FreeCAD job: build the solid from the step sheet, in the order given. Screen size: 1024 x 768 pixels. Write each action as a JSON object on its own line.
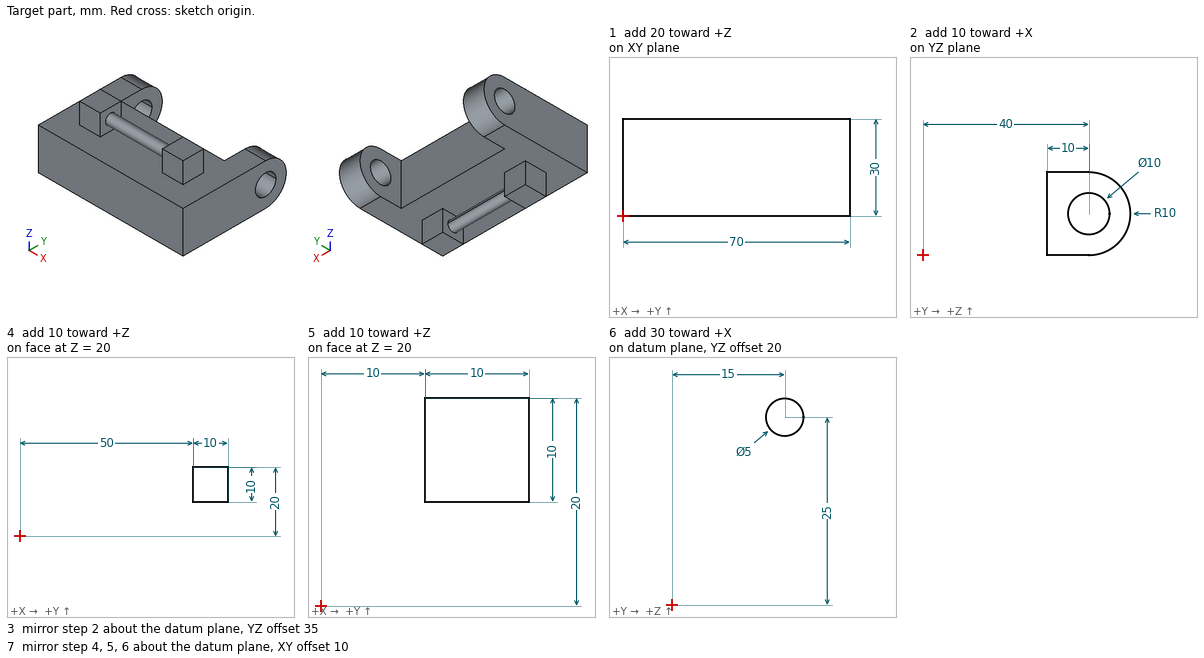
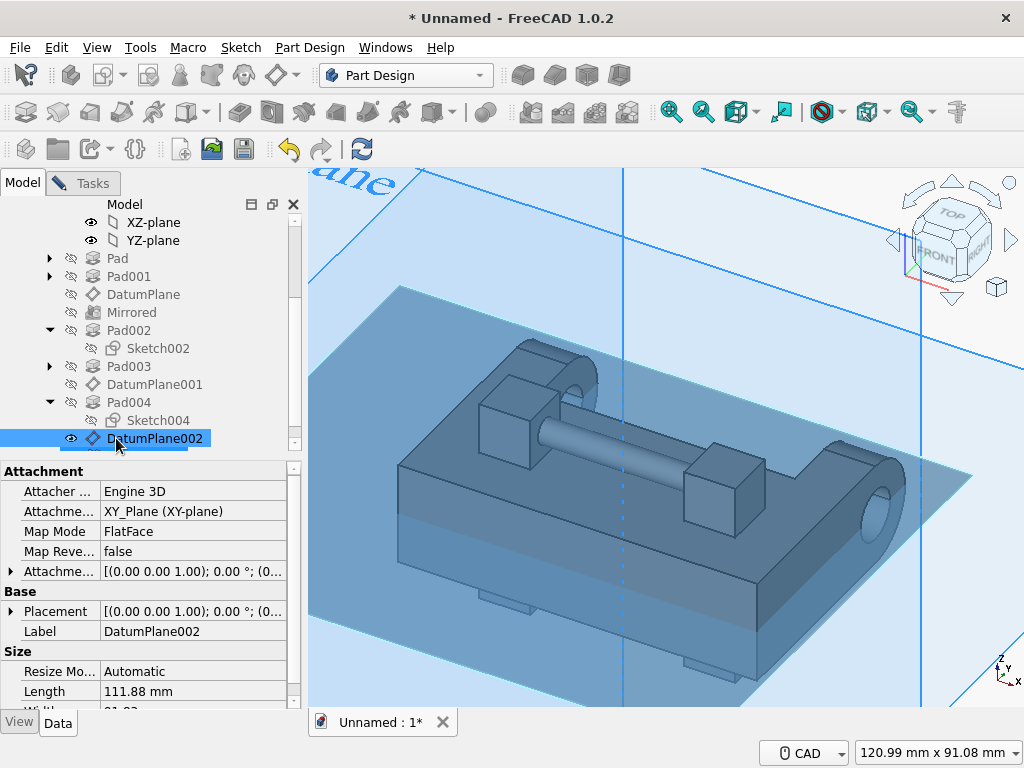
{"action": "left_click", "coordinate": [84, 182]}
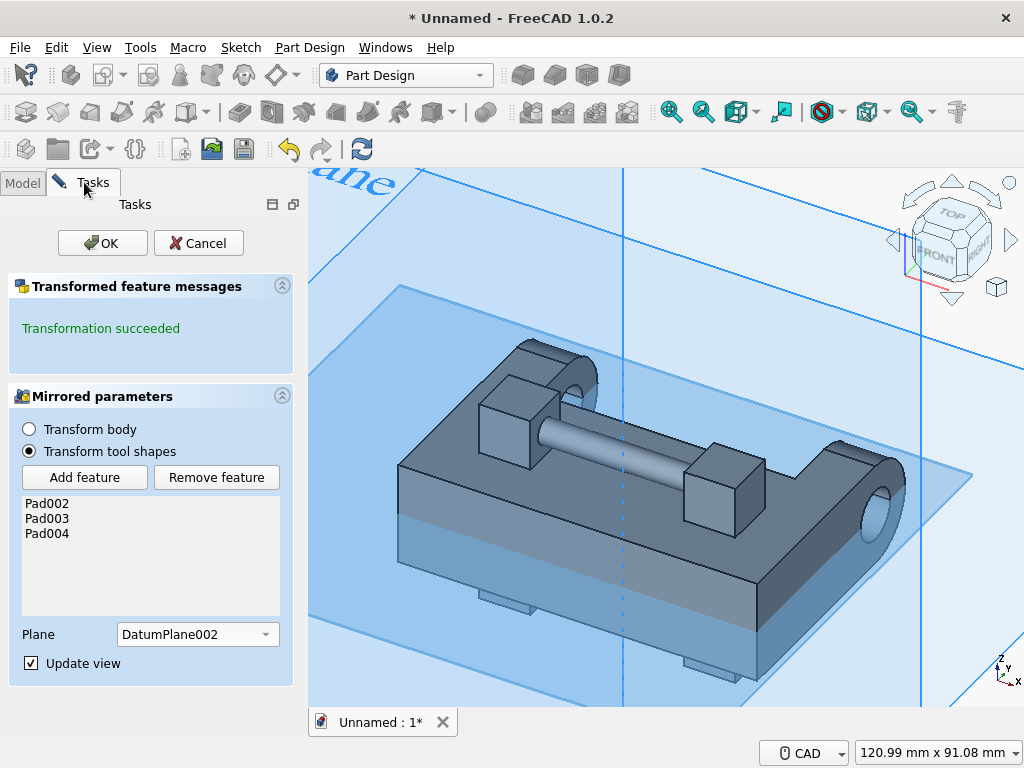
{"action": "left_click", "coordinate": [103, 243]}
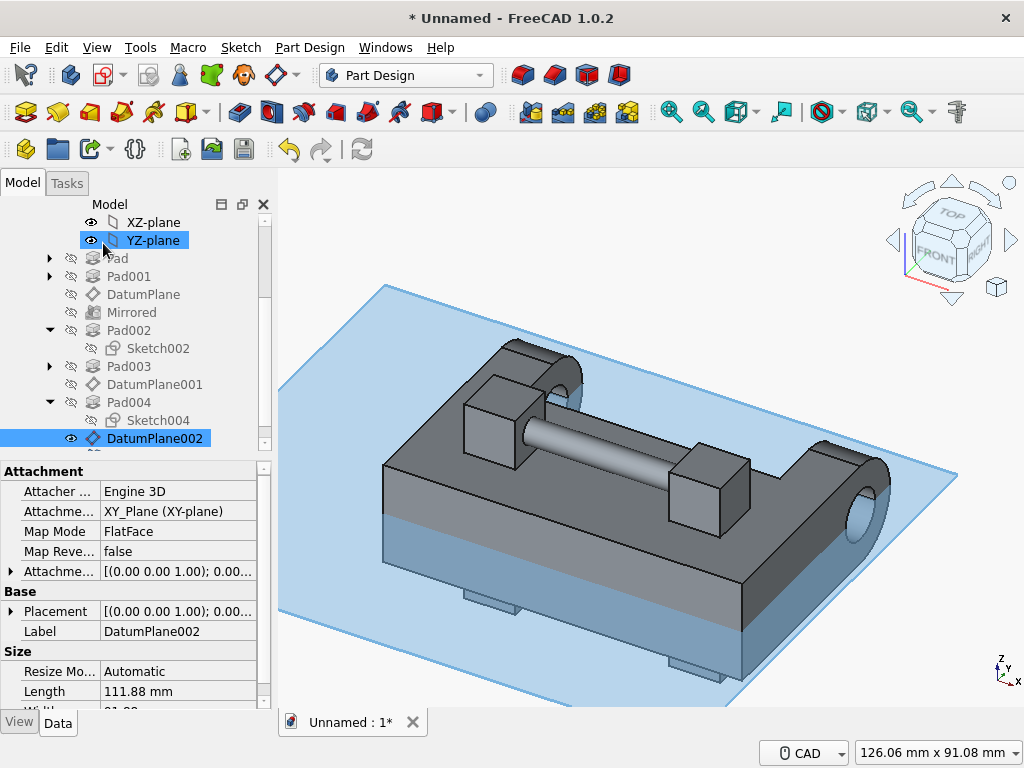
{"action": "left_click", "coordinate": [116, 438]}
{"action": "key", "text": "space"}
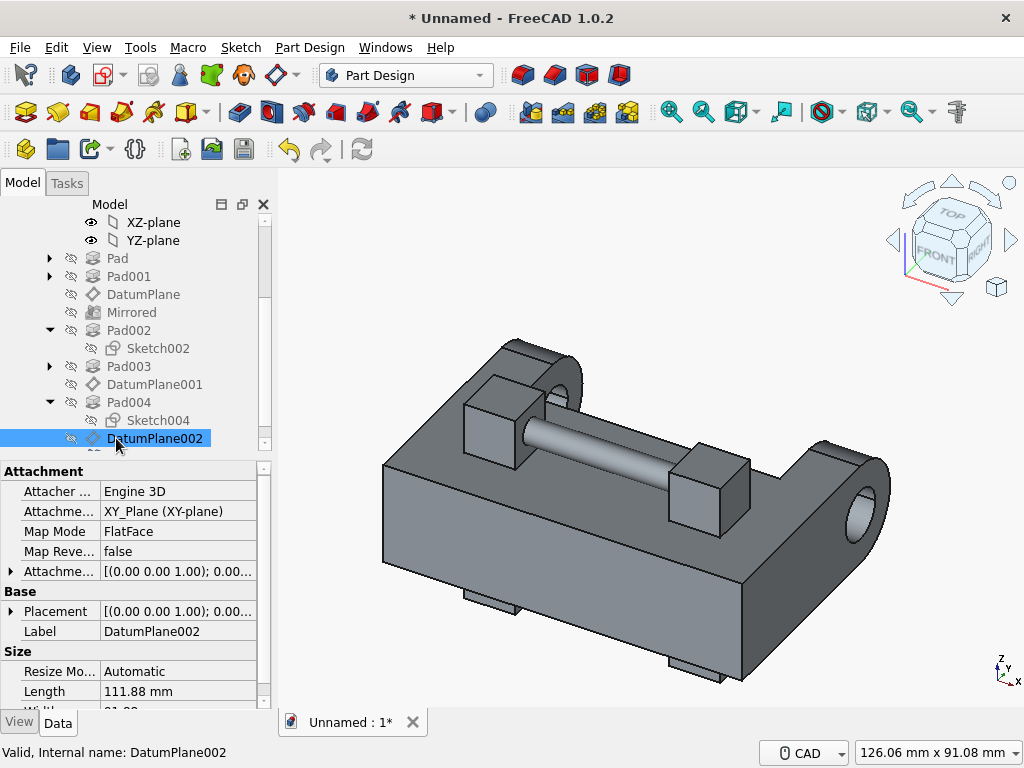
{"action": "key", "text": "0"}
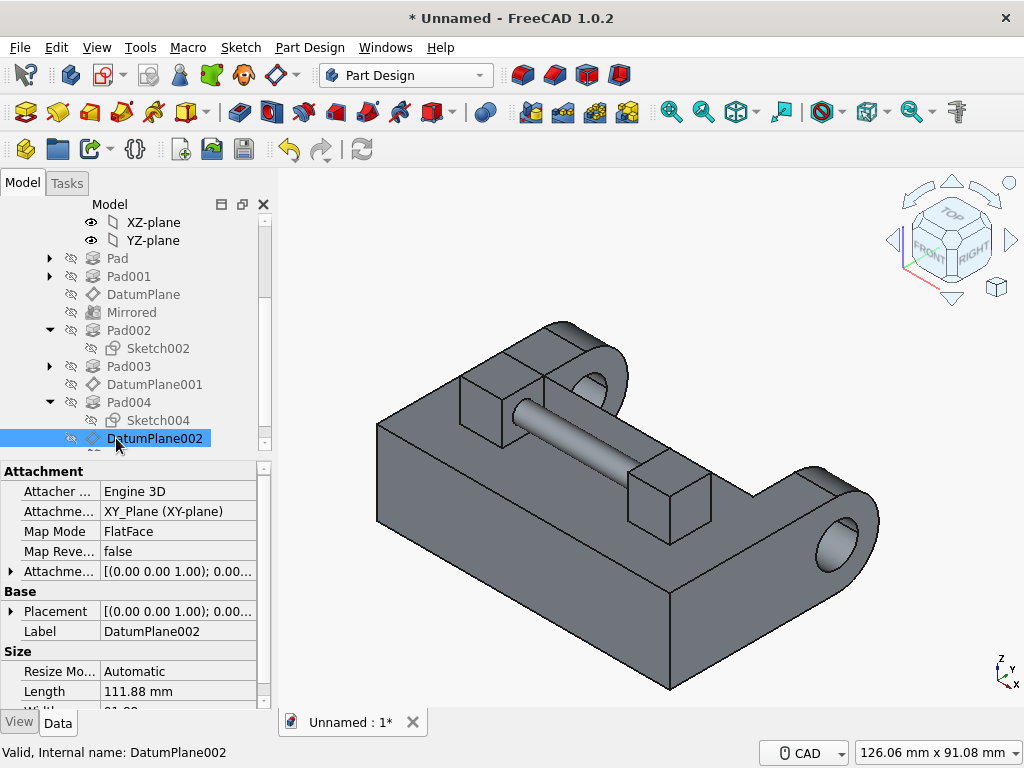
{"action": "key", "text": "v f"}